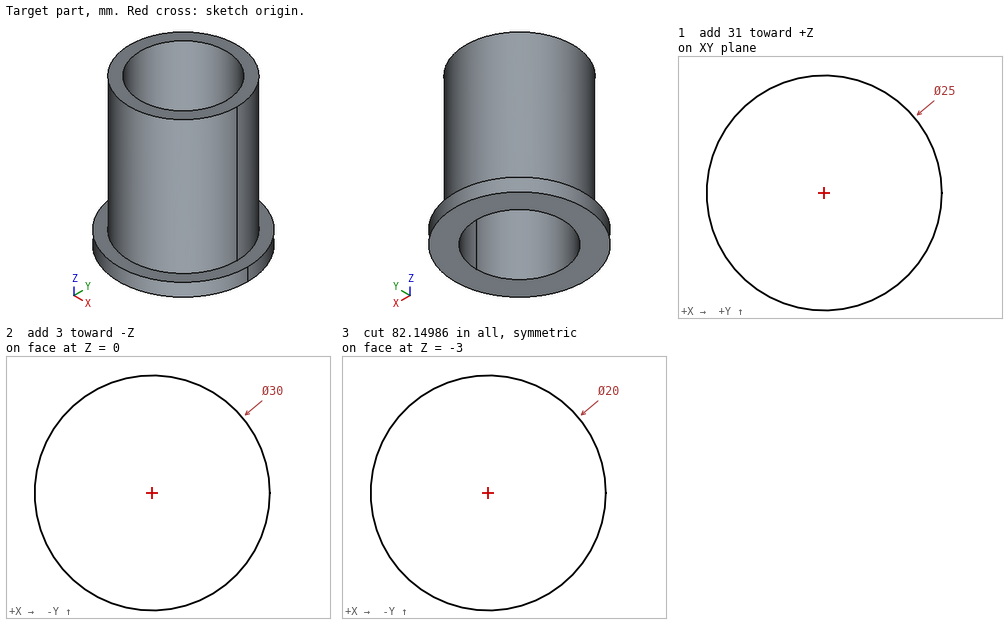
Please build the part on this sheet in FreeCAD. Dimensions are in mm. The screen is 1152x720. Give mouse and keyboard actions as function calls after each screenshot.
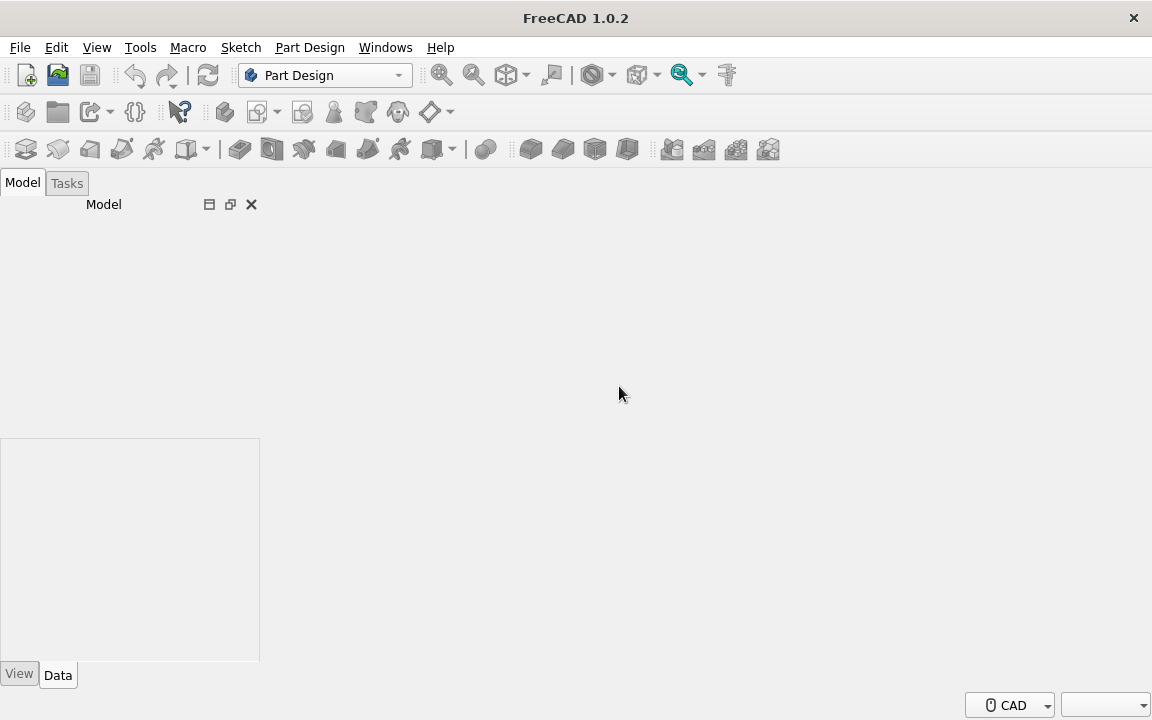
click(26, 76)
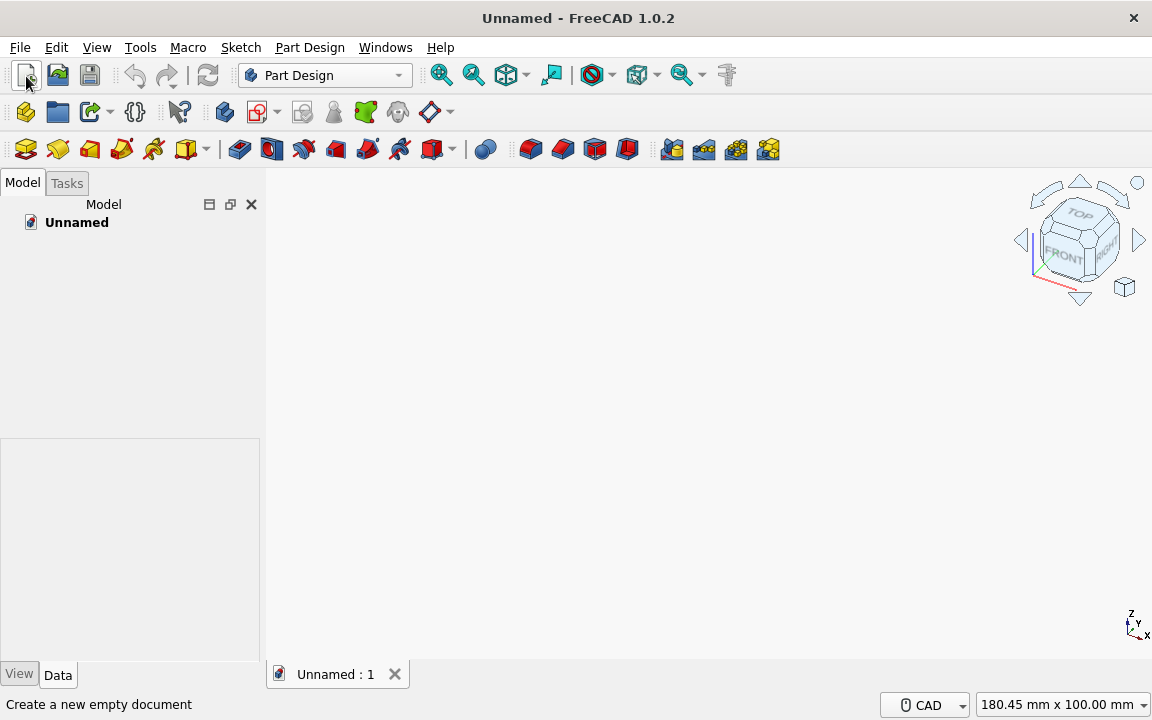
click(258, 112)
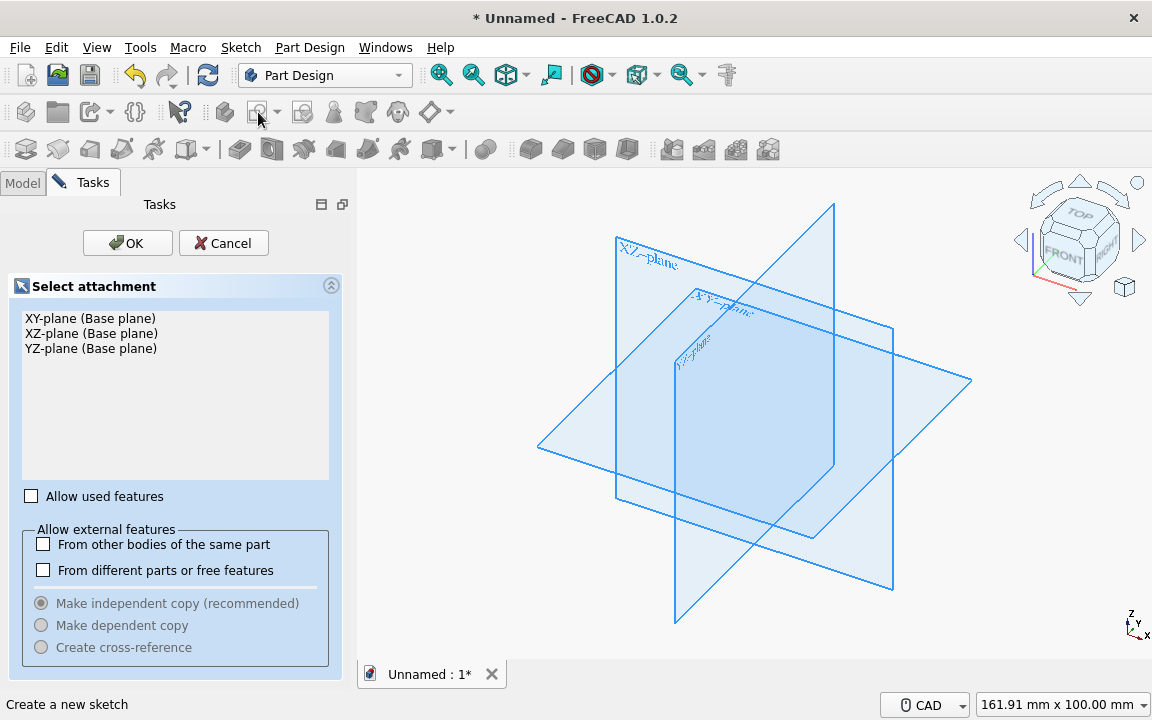
click(82, 318)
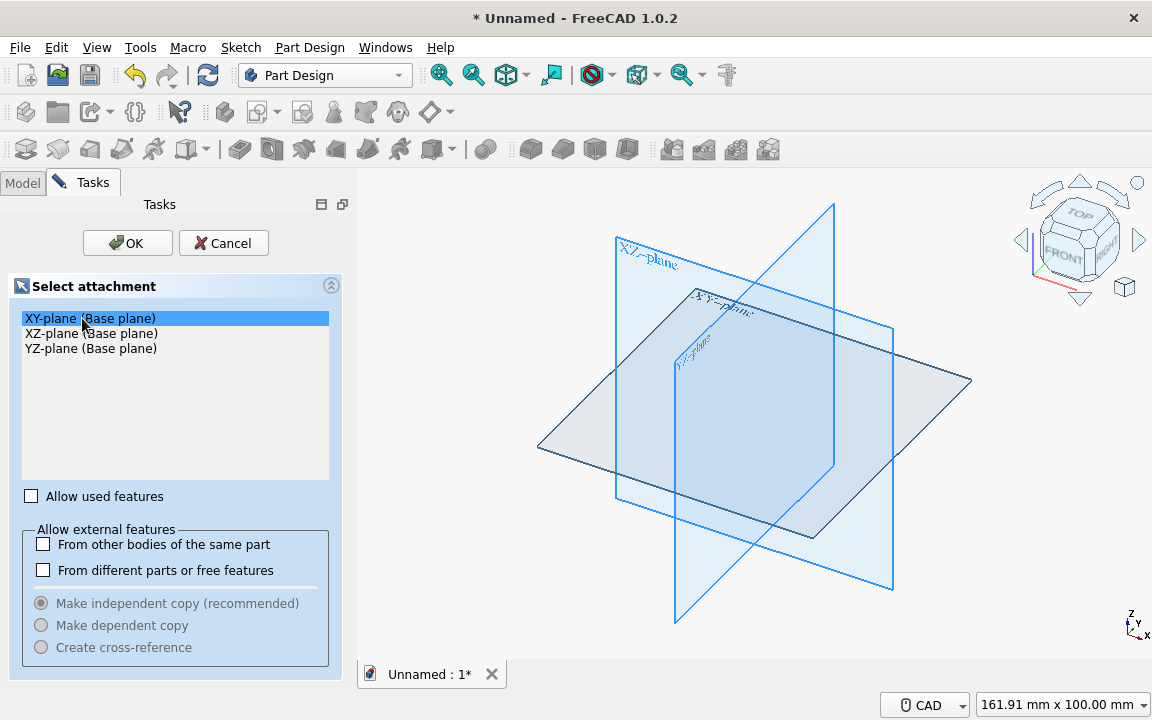
click(128, 243)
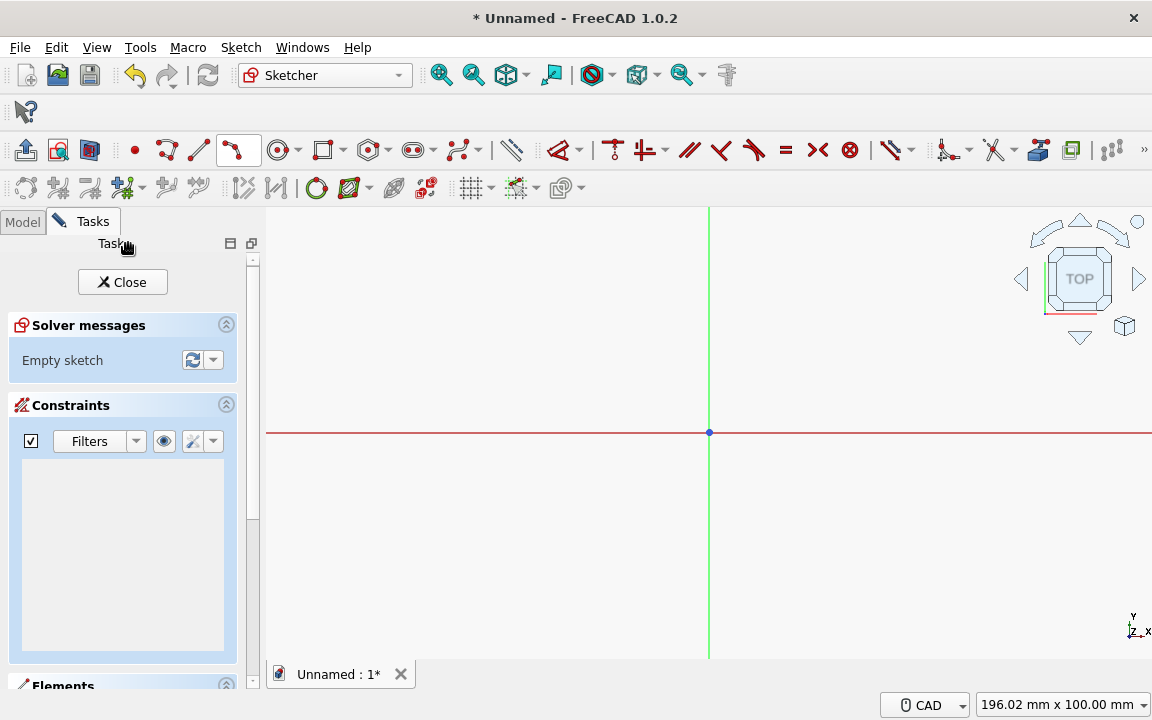
scroll(749, 433, up, 5)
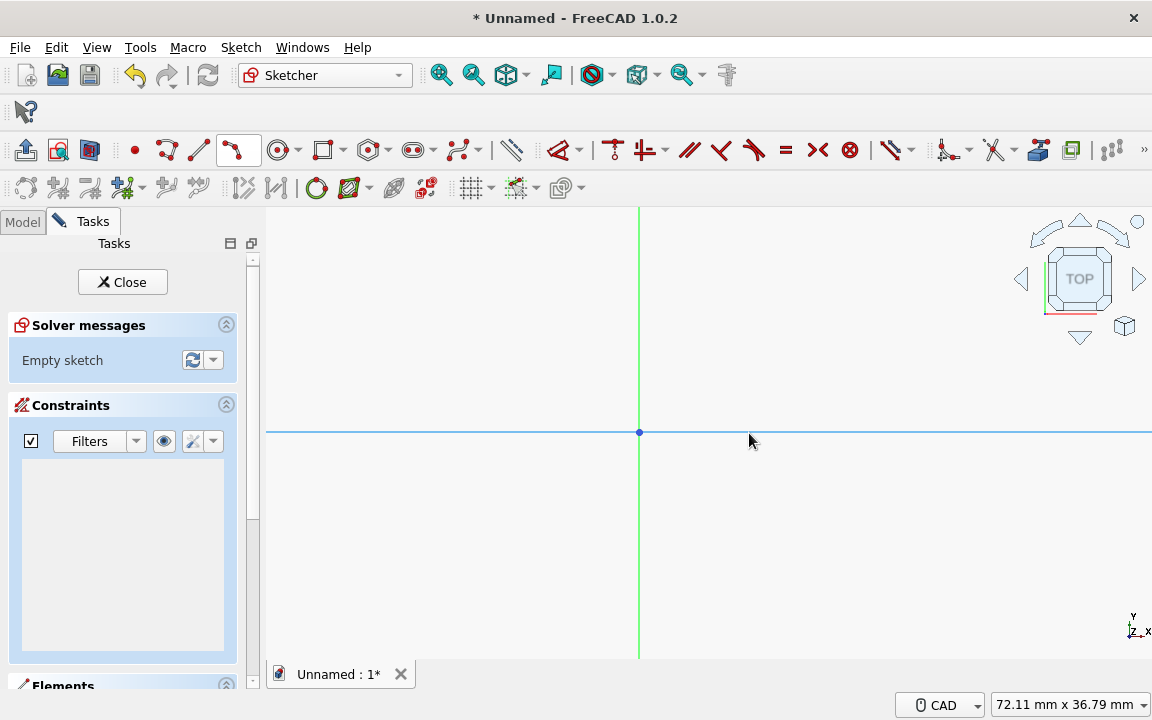
click(278, 150)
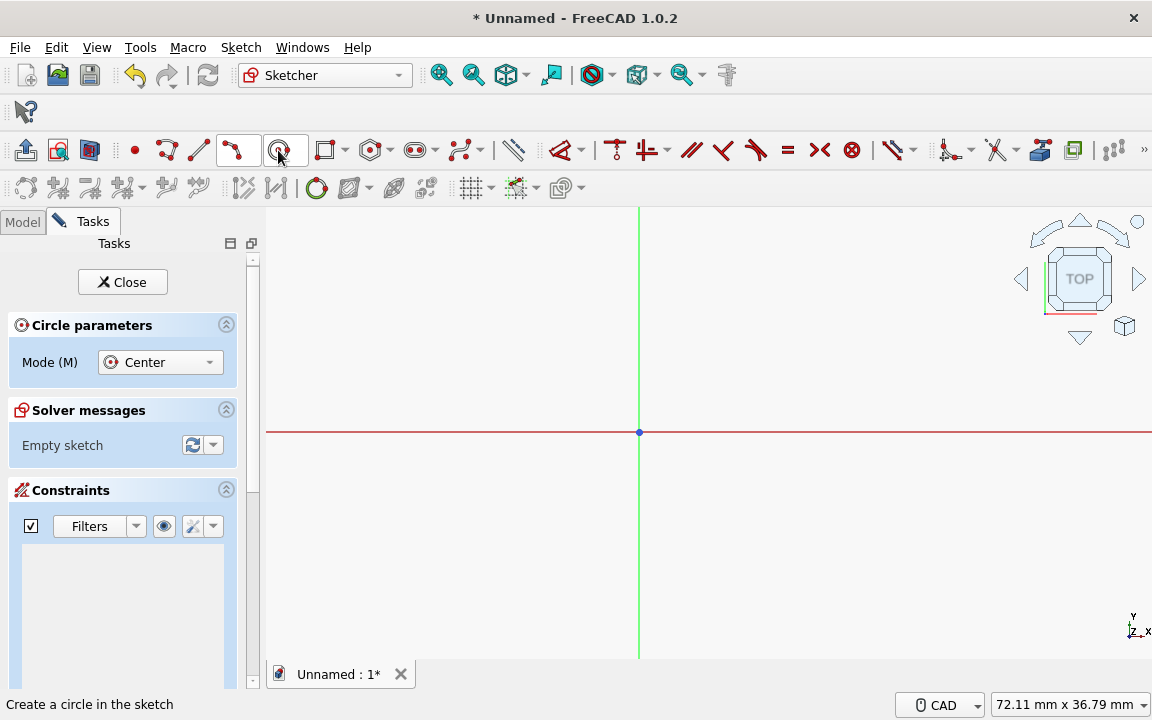
click(639, 432)
click(748, 324)
key(Escape)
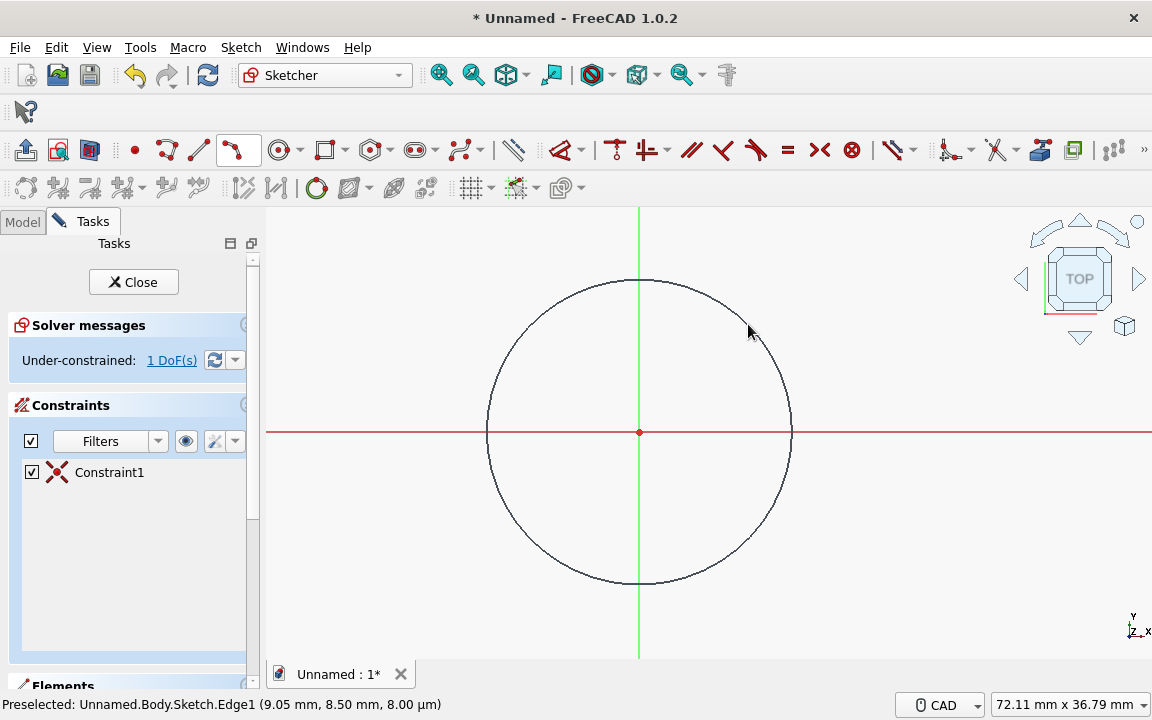
click(560, 150)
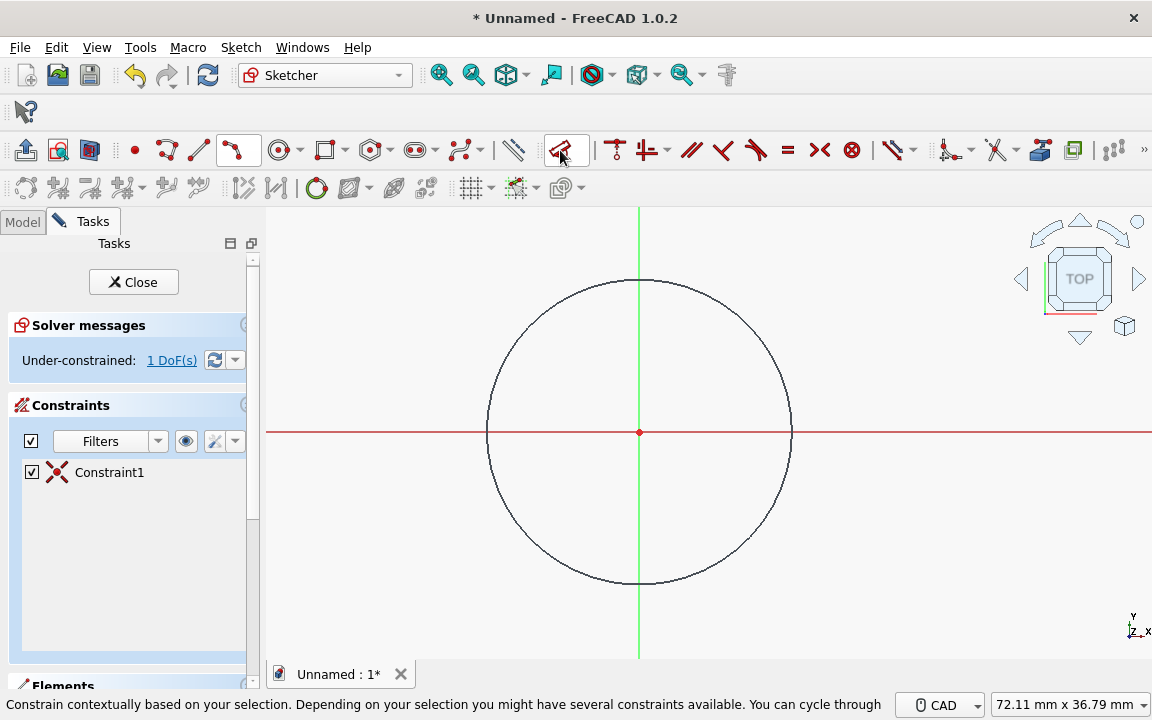
click(747, 324)
click(770, 301)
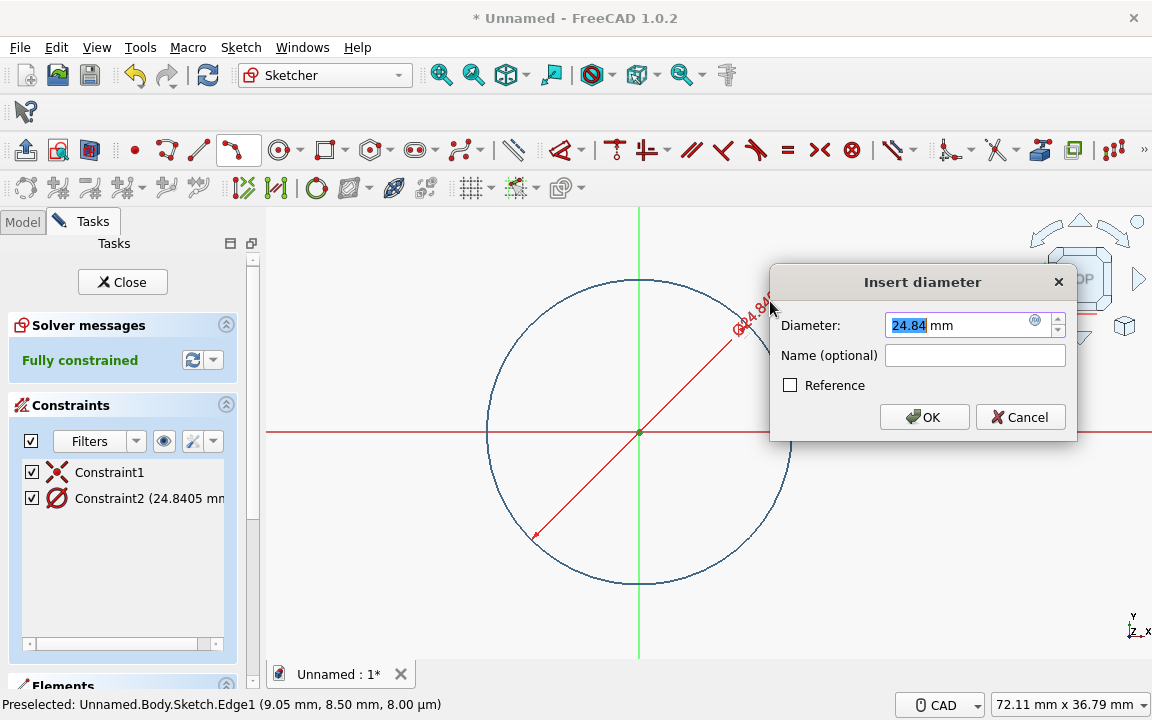
text(25)
key(Return)
key(Escape)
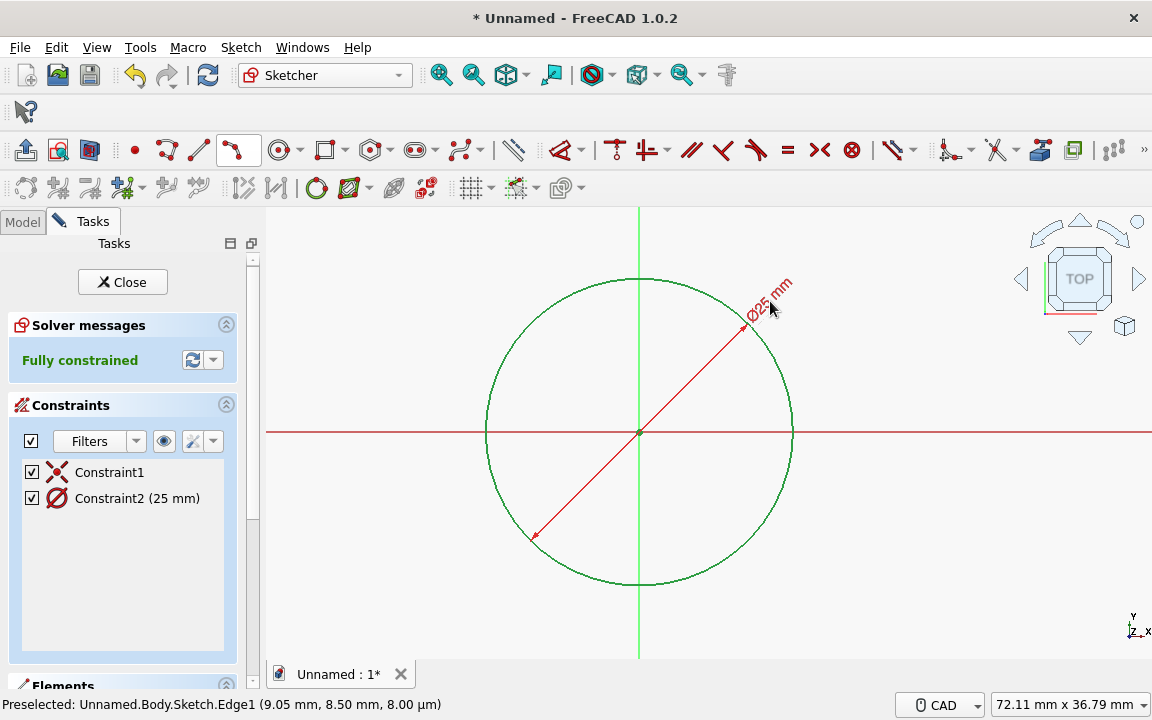
click(123, 282)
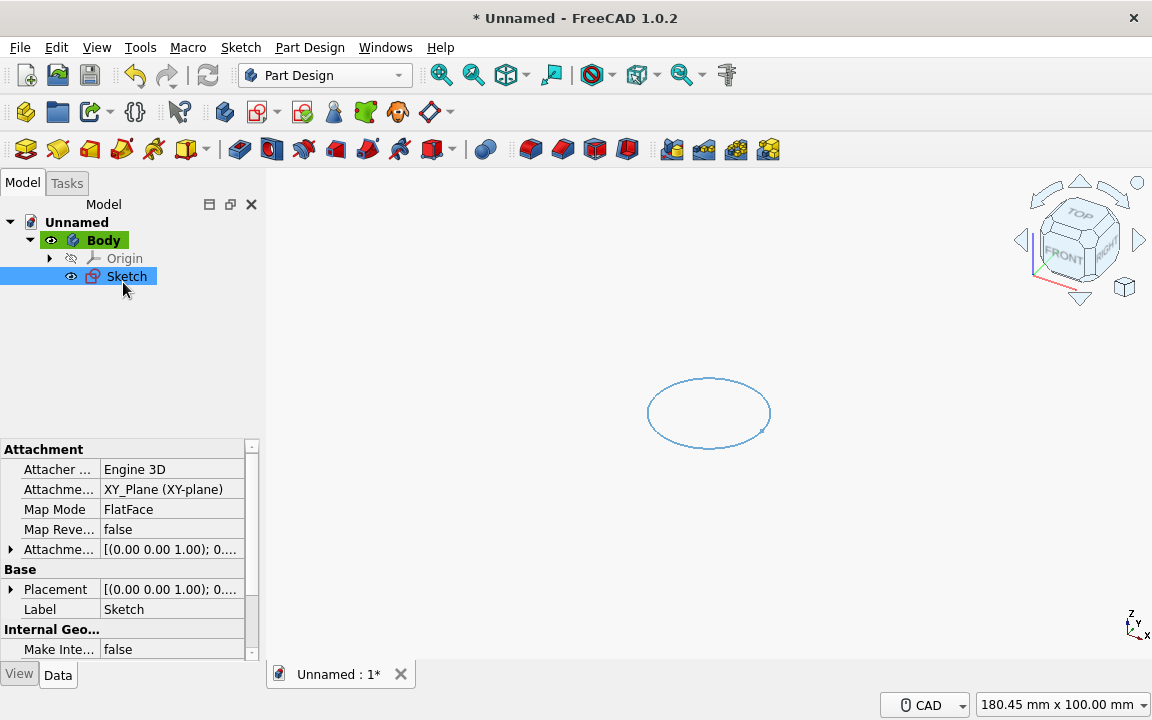
click(26, 150)